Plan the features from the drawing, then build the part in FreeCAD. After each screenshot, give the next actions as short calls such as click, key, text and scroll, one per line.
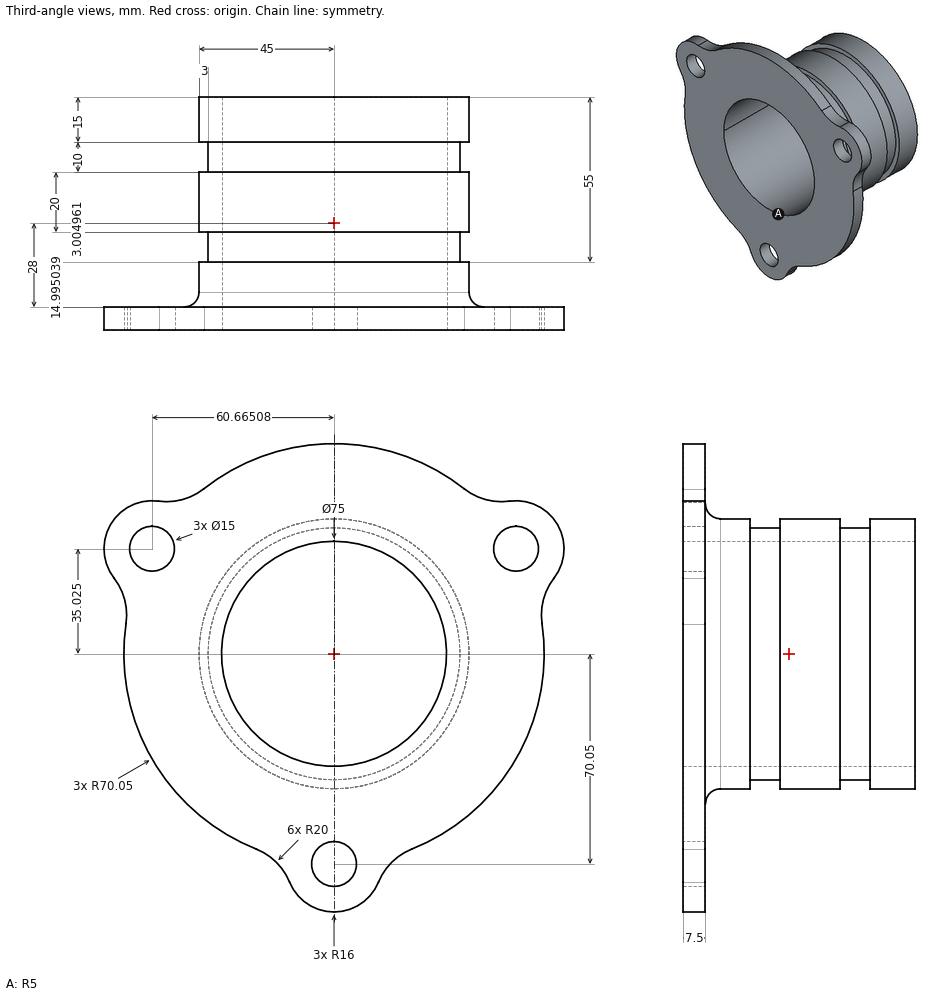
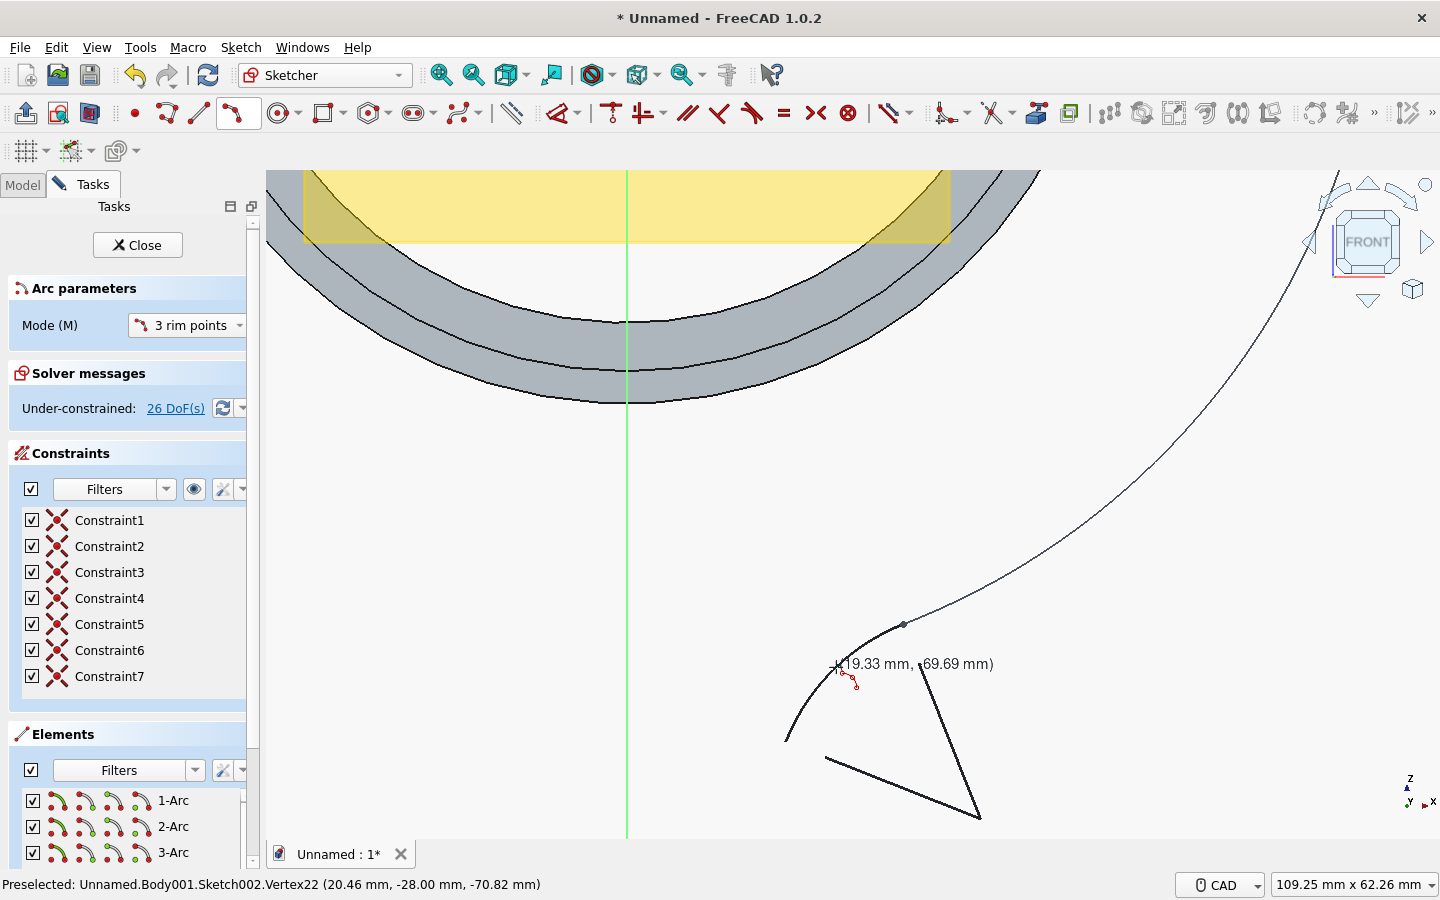
click(834, 666)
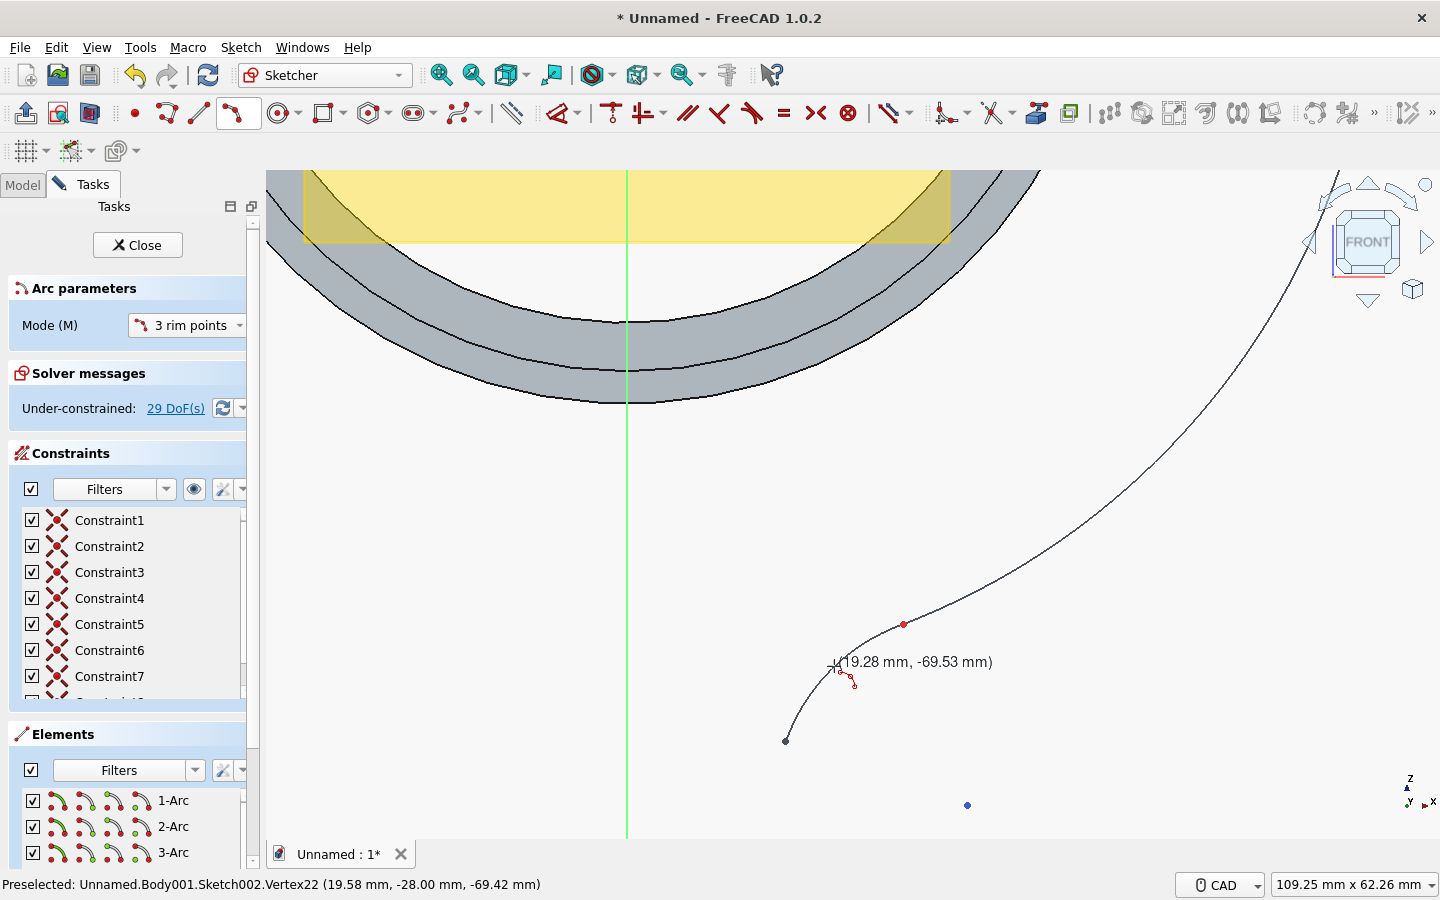
scroll(836, 668, down, 7)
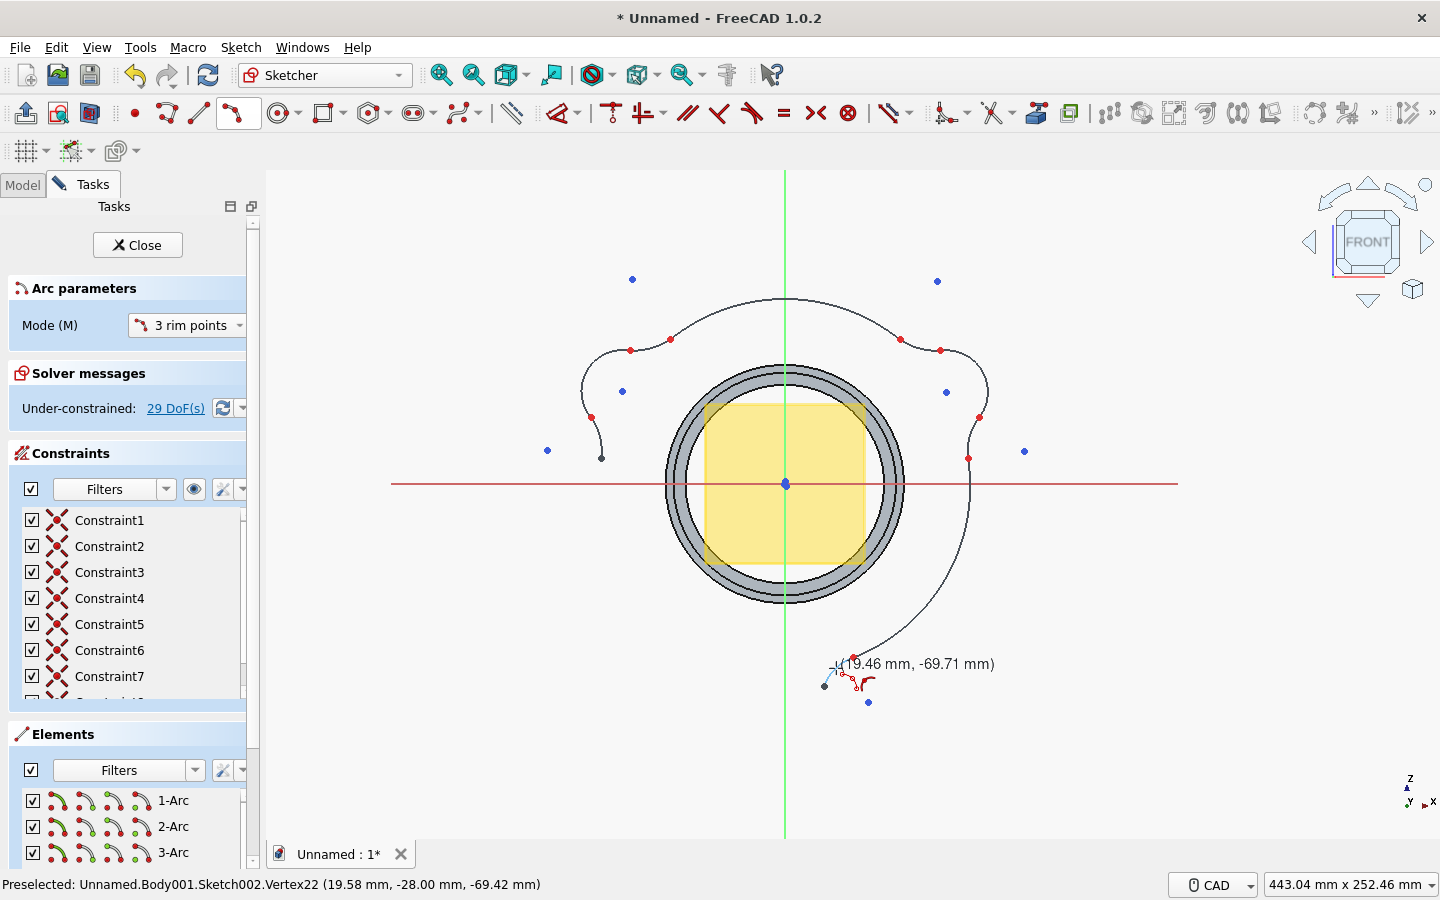
click(824, 687)
click(746, 686)
click(765, 707)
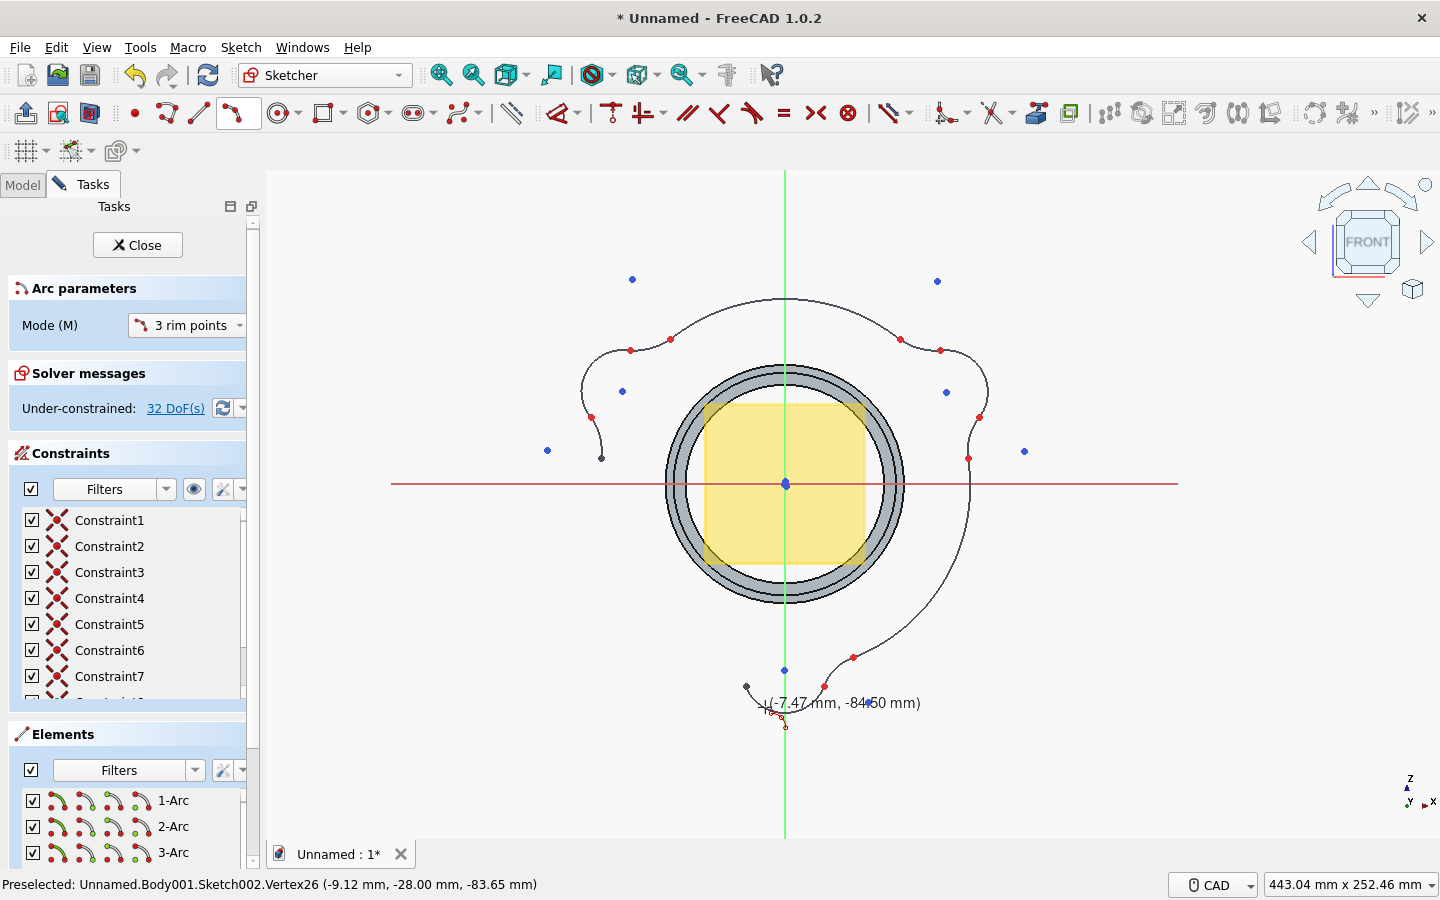
click(746, 687)
click(716, 657)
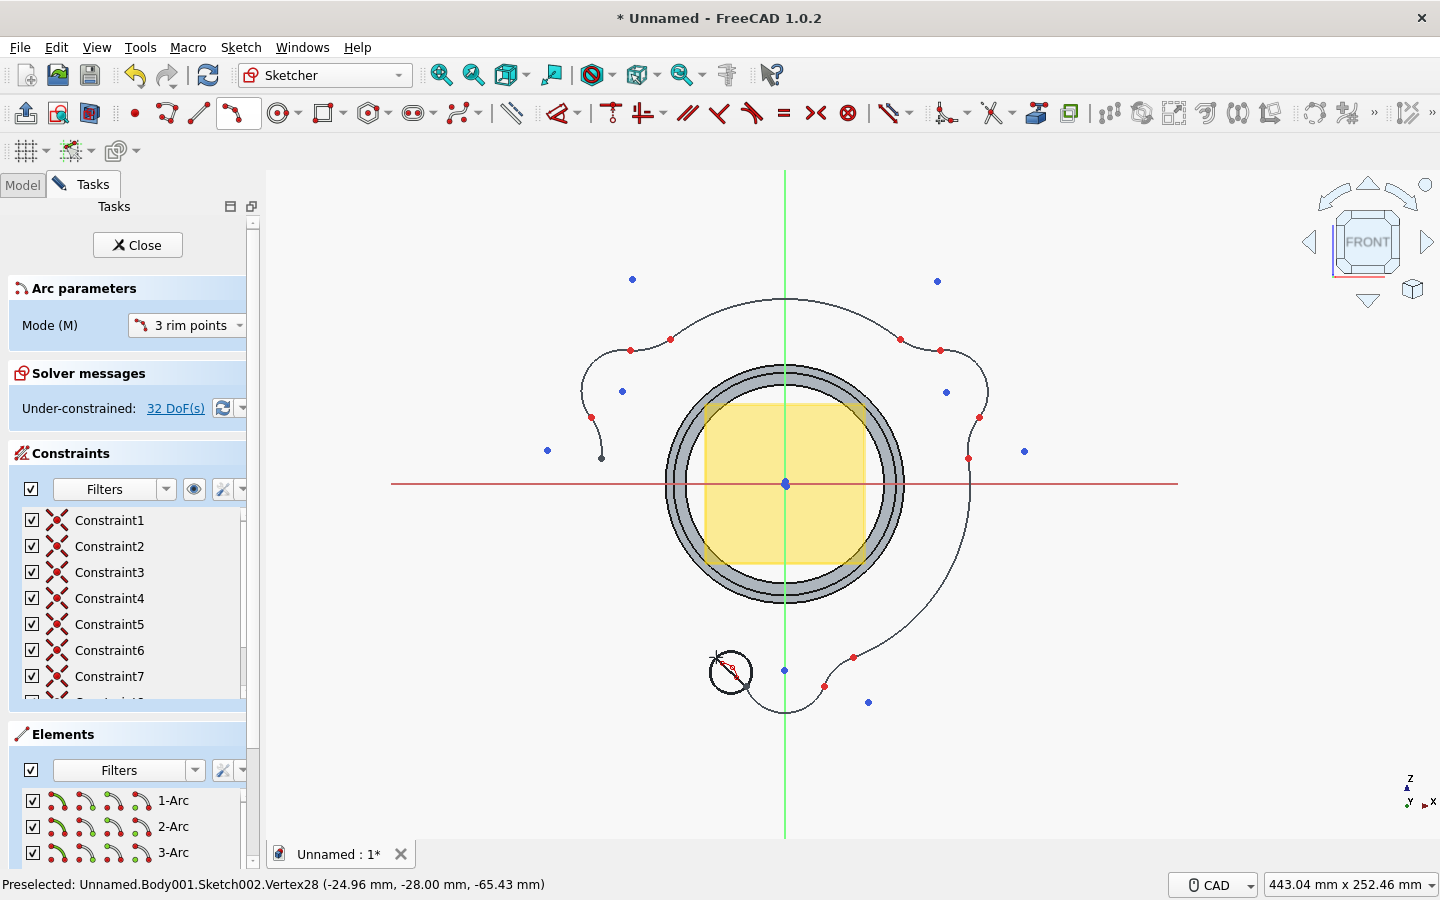
scroll(734, 668, up, 7)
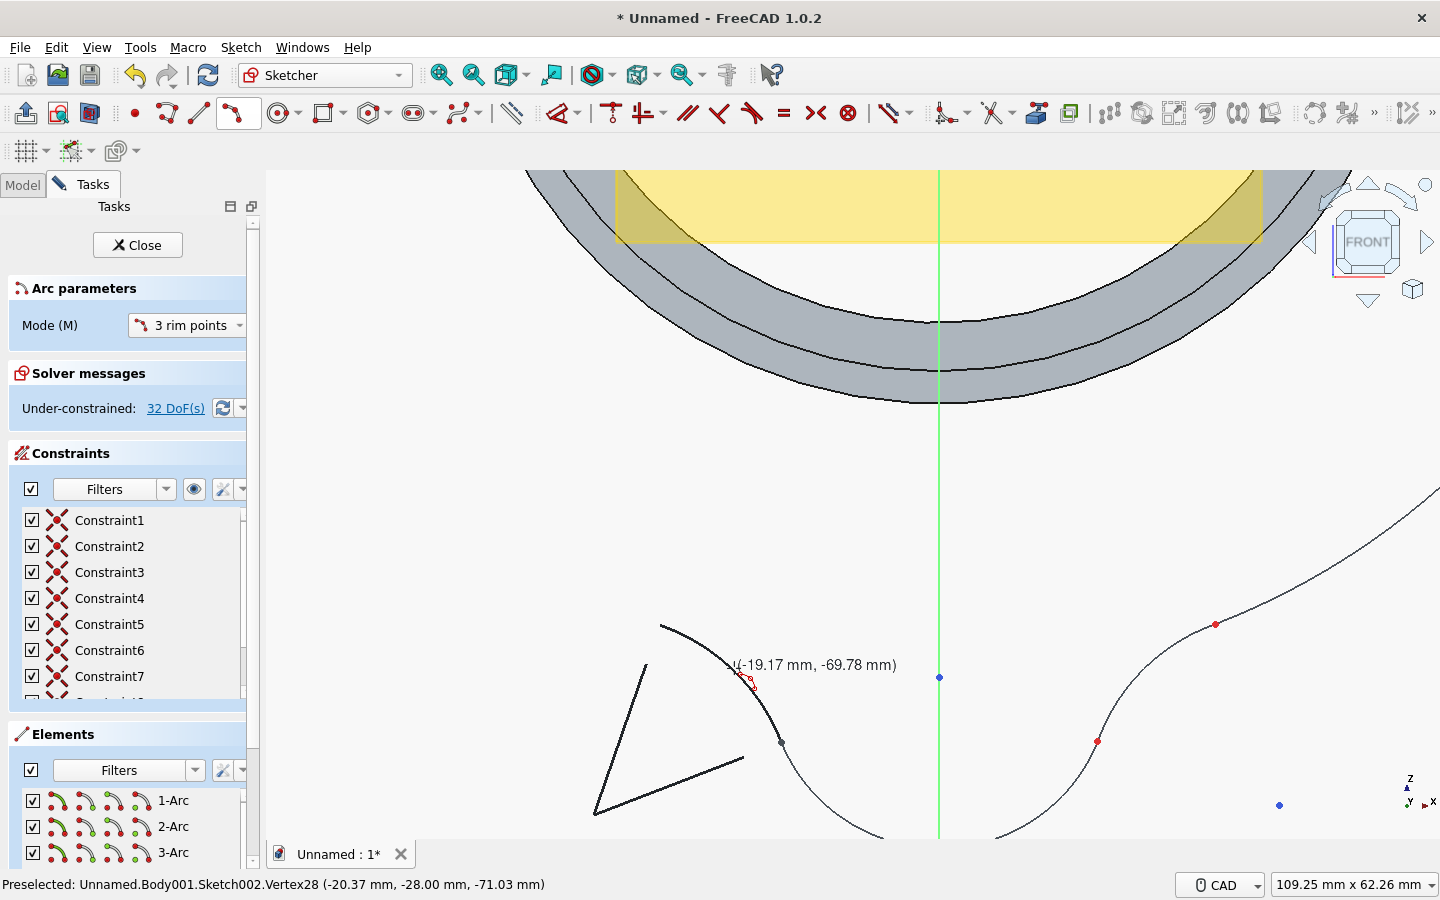
click(732, 666)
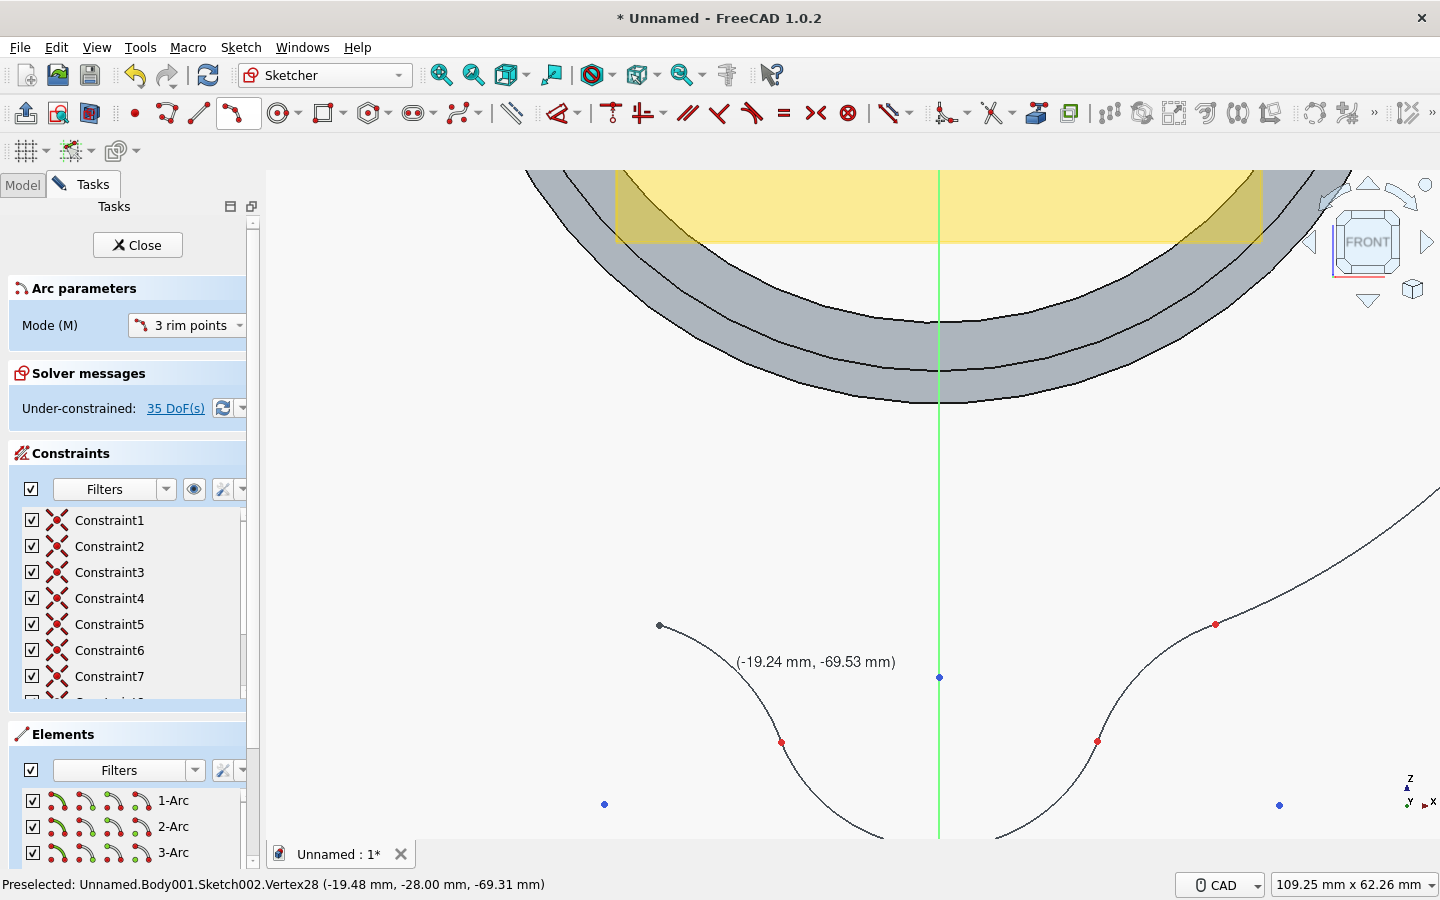
scroll(734, 668, down, 7)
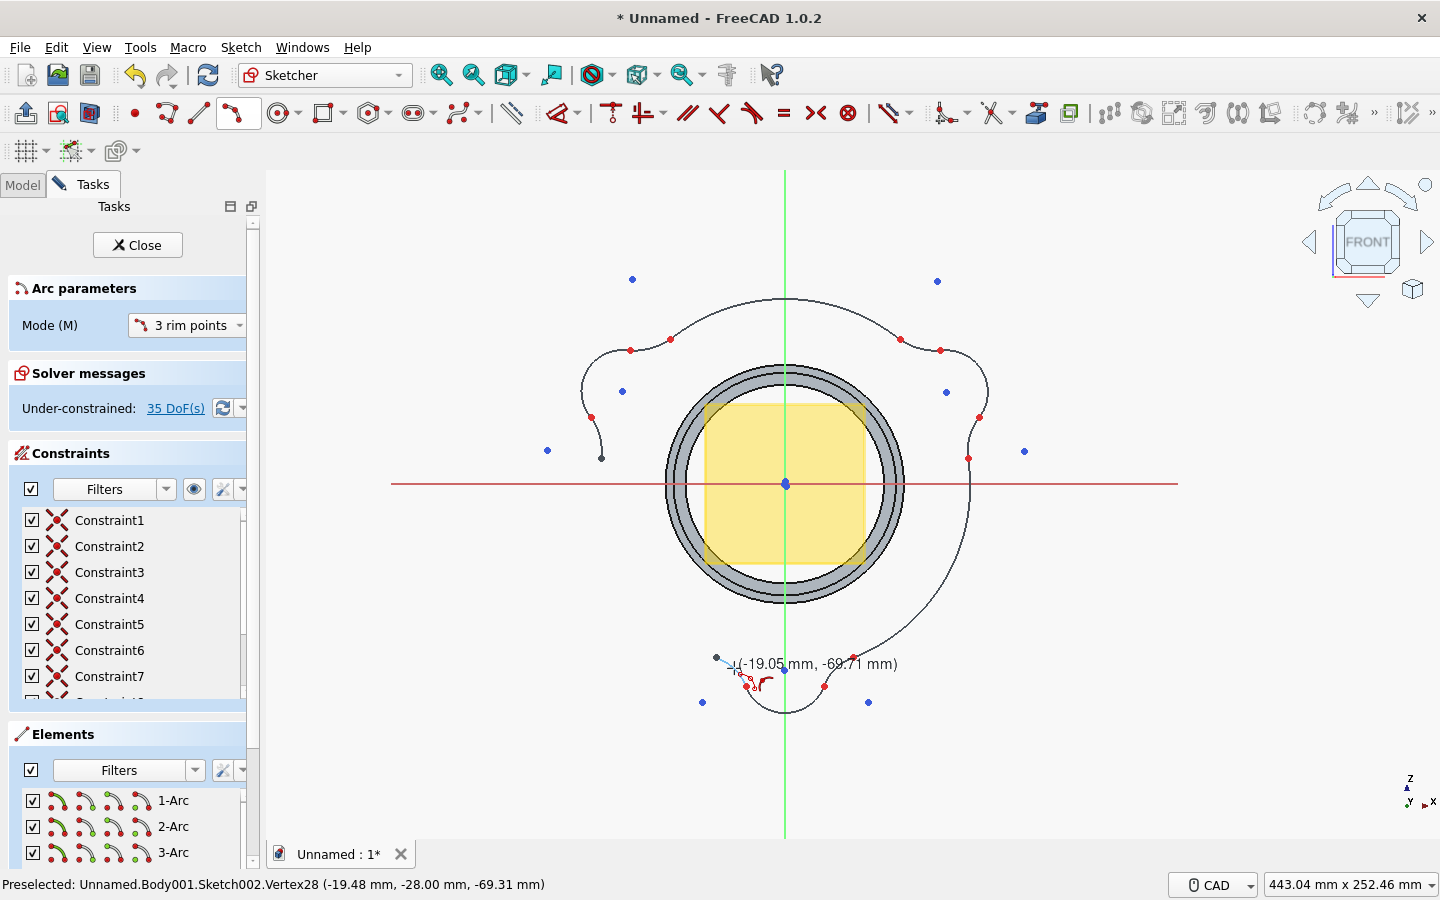
click(716, 658)
click(601, 459)
click(624, 577)